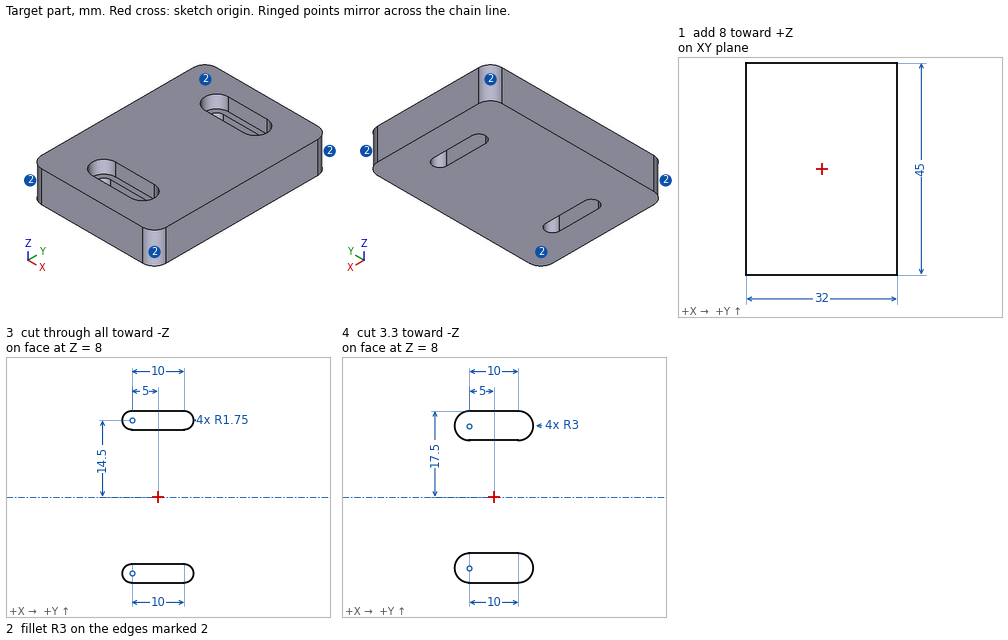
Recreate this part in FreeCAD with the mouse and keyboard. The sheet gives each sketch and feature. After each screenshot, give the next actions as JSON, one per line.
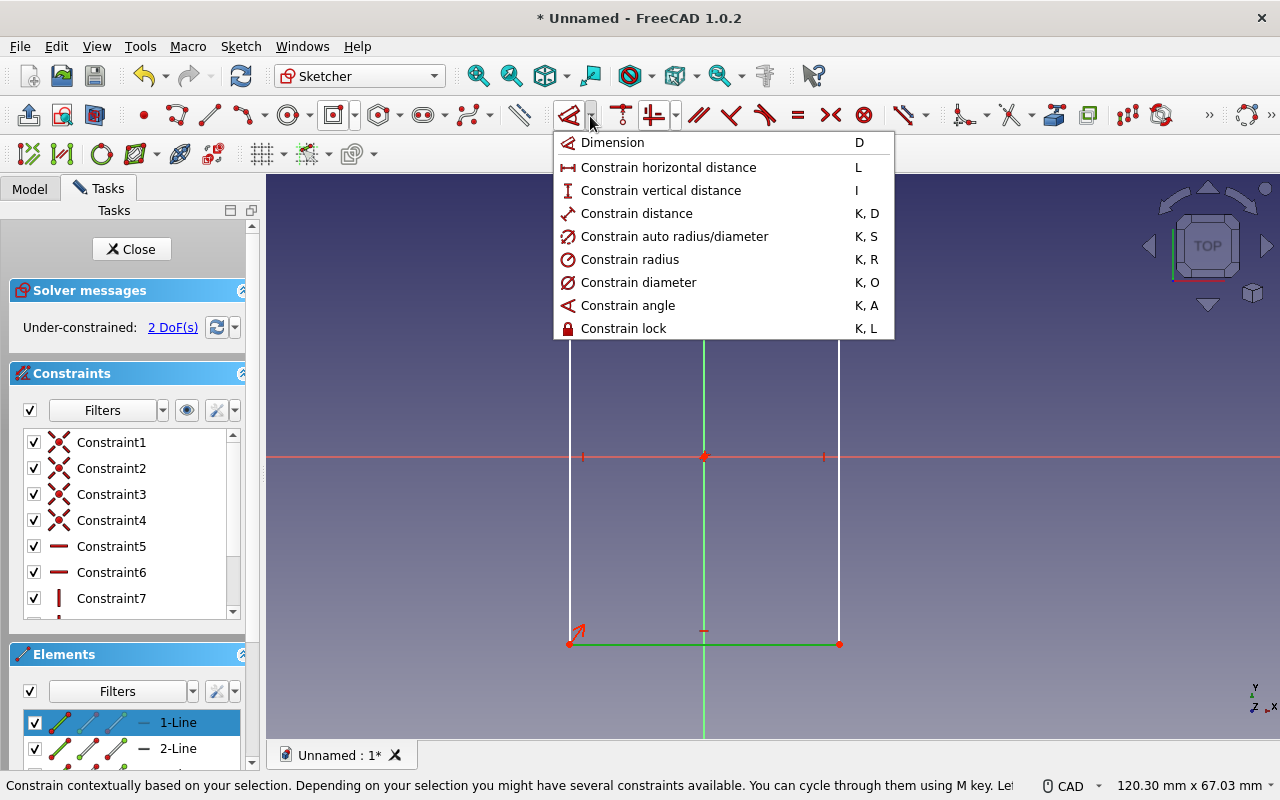
{"action": "left_click", "coordinate": [724, 168]}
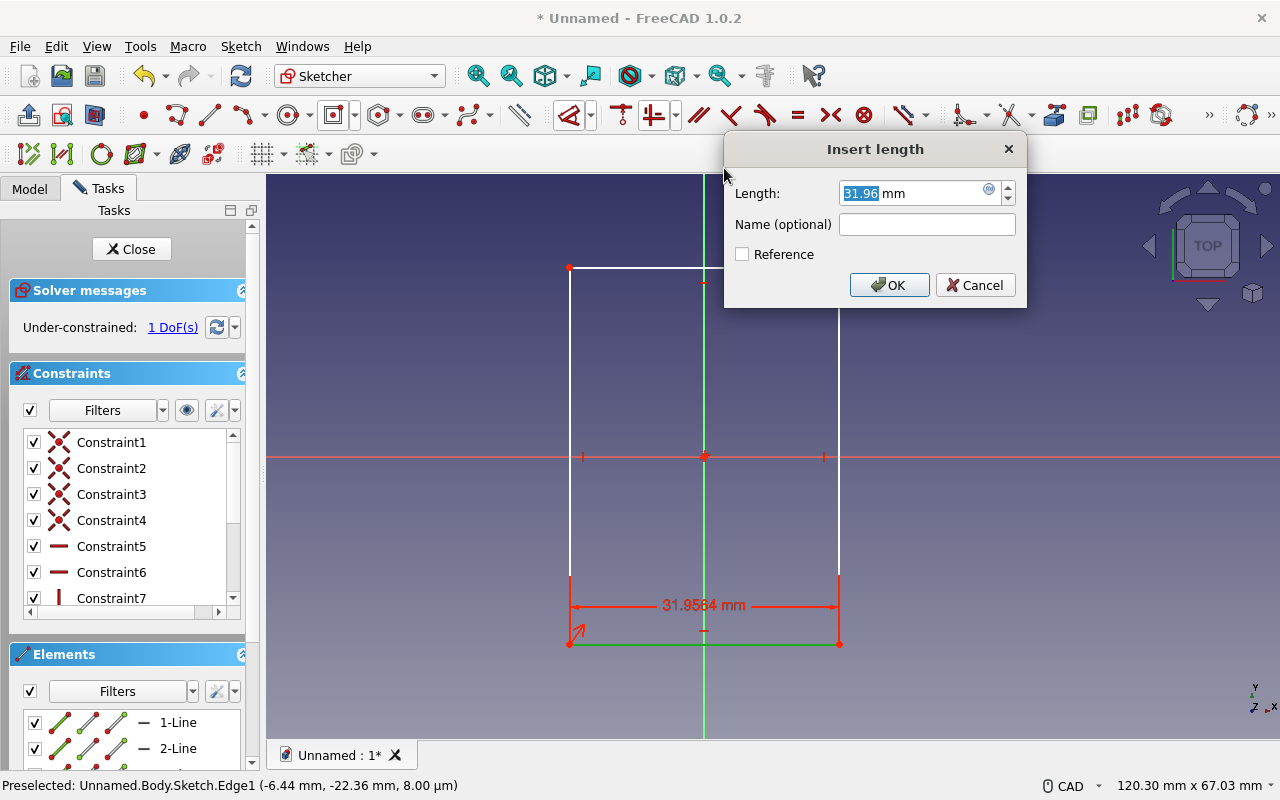
{"action": "type", "text": "32"}
{"action": "key", "text": "Return"}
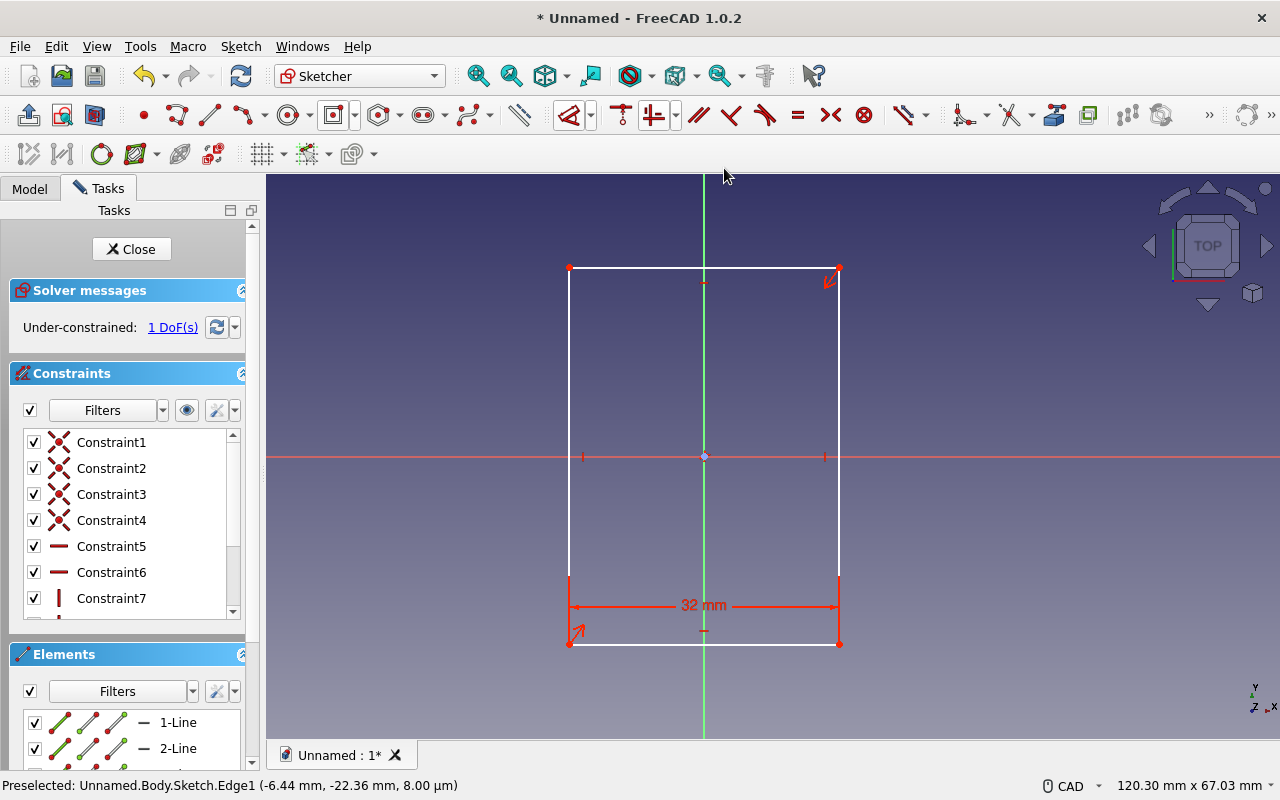
{"action": "left_click", "coordinate": [839, 532]}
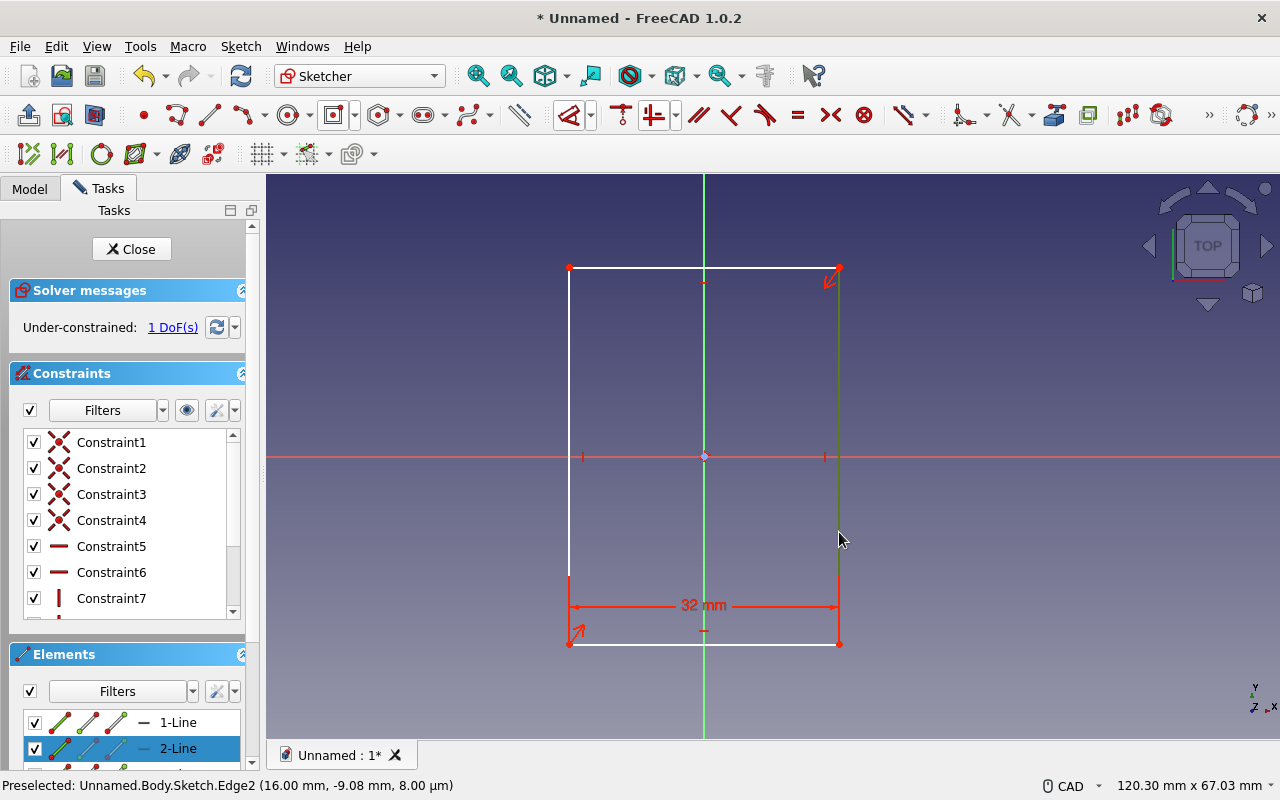
{"action": "left_click", "coordinate": [590, 116]}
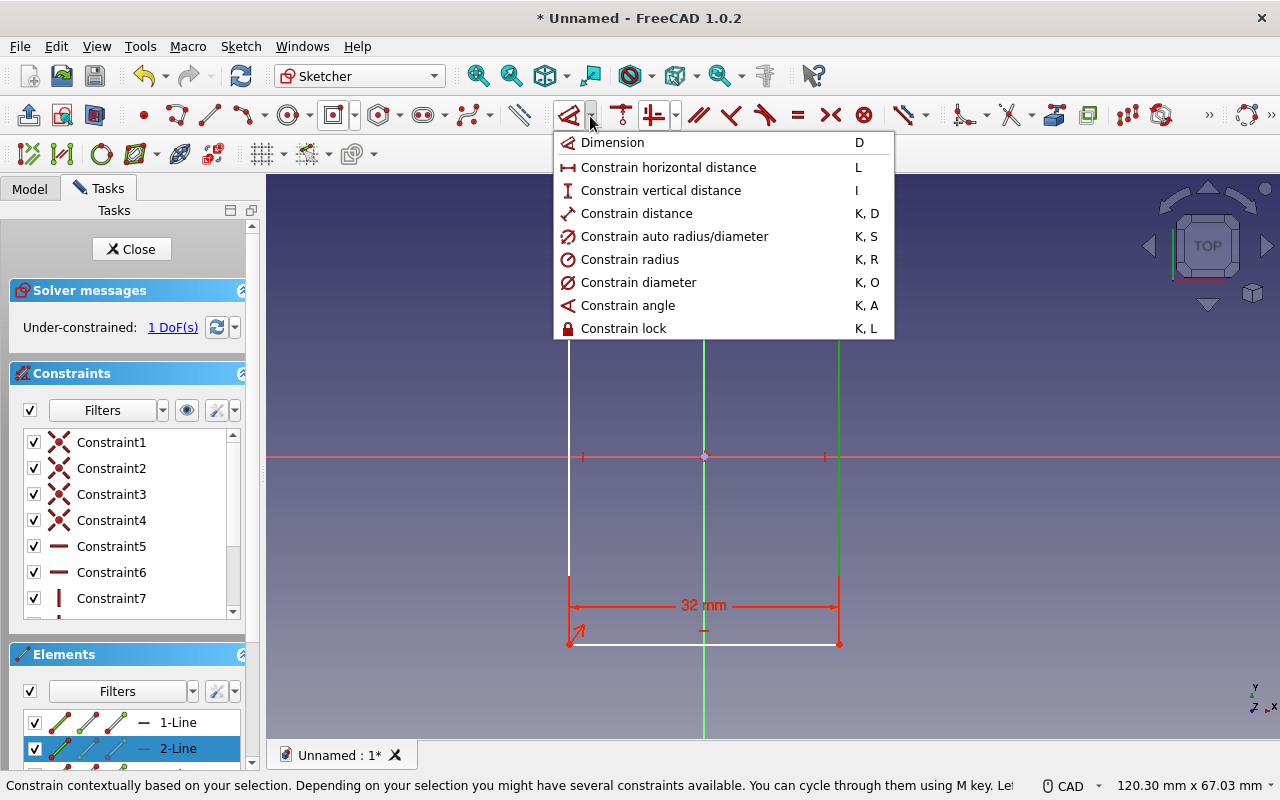
{"action": "left_click", "coordinate": [724, 190]}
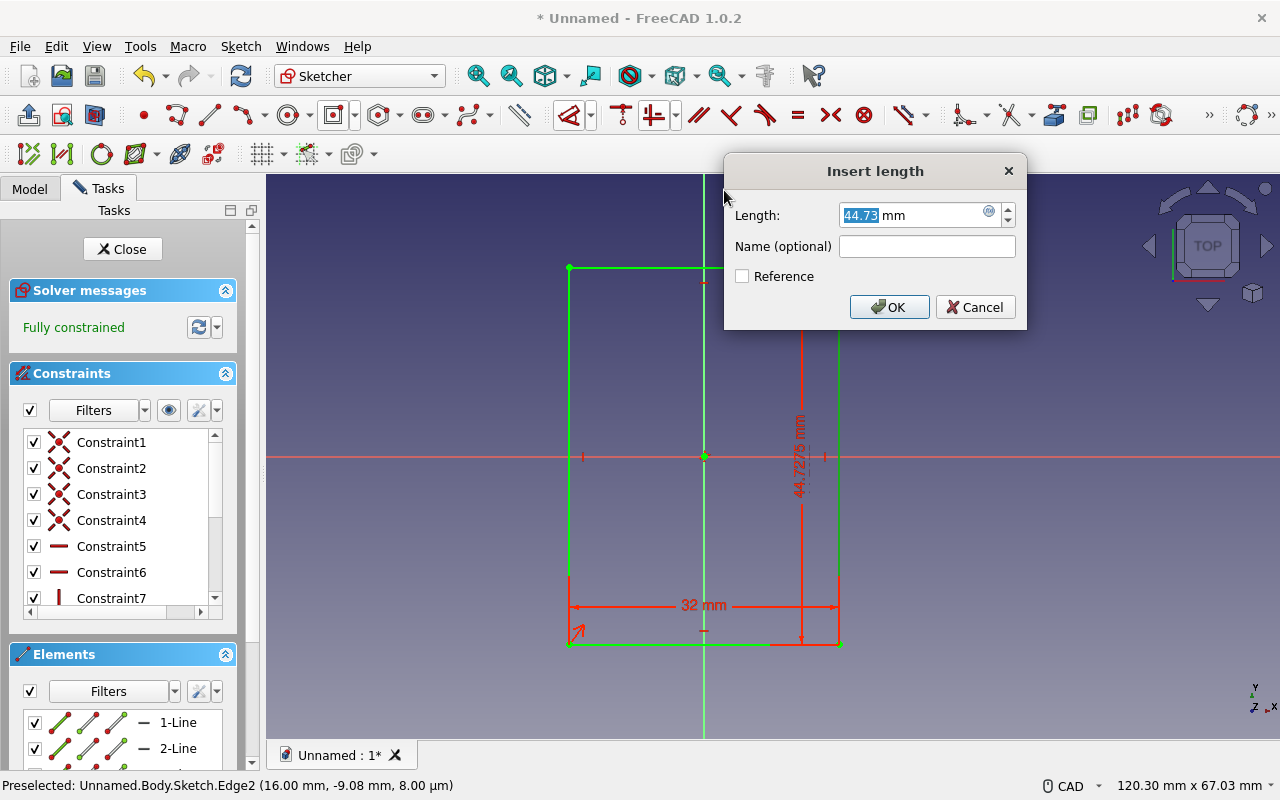
{"action": "type", "text": "45"}
{"action": "key", "text": "Return"}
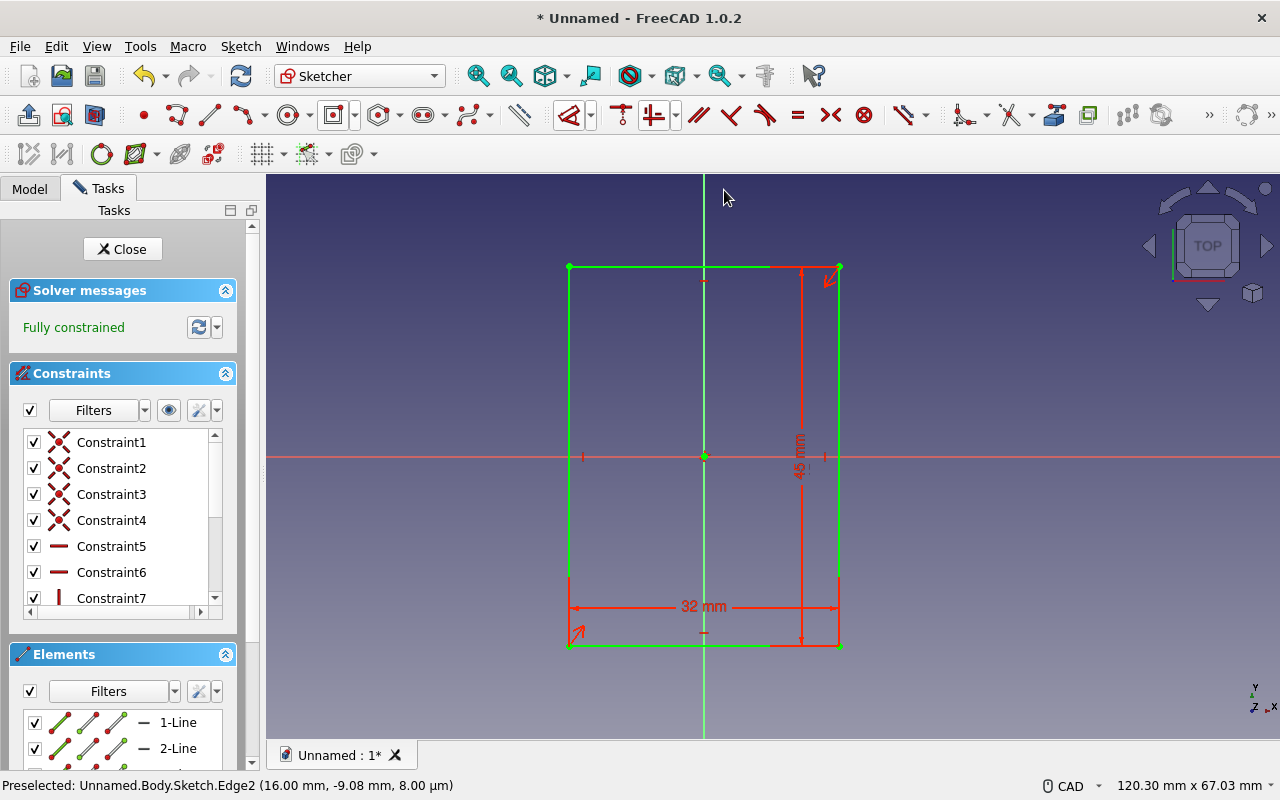
{"action": "left_click", "coordinate": [123, 249]}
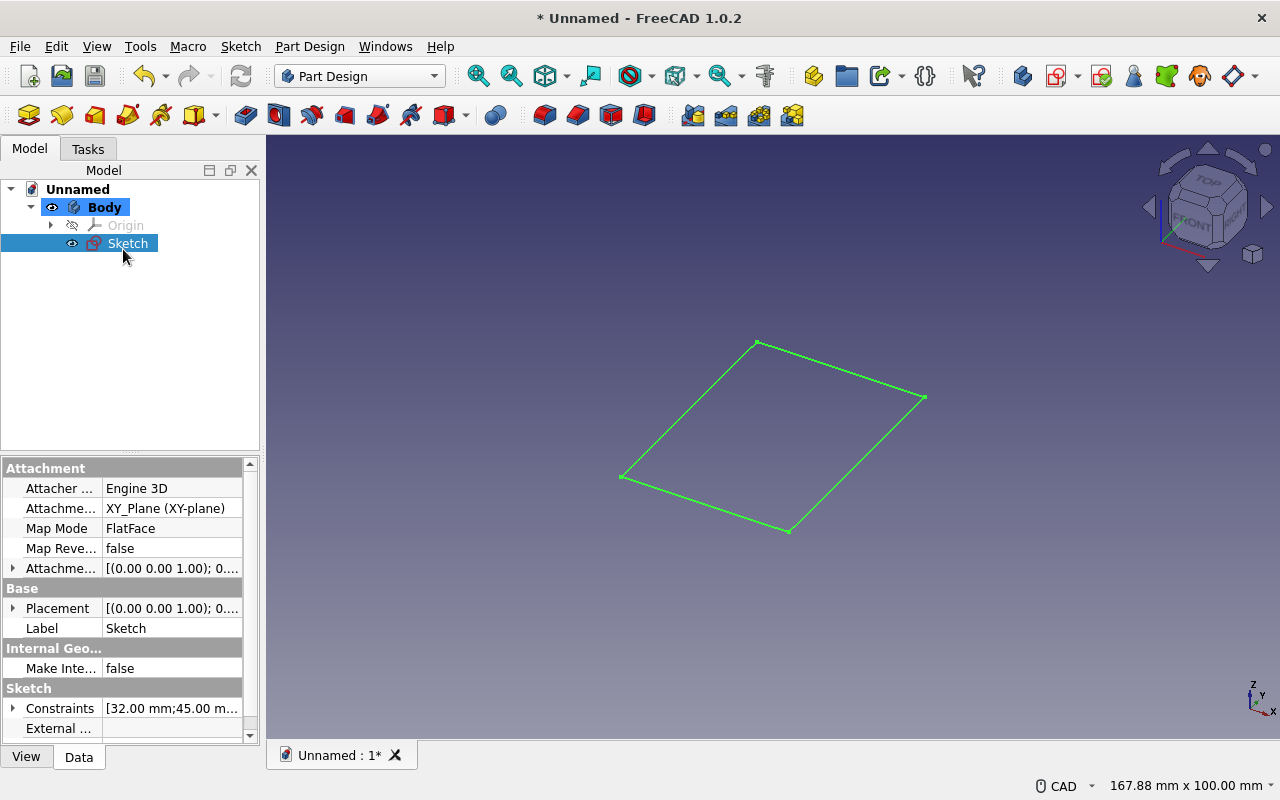
{"action": "left_click", "coordinate": [29, 116]}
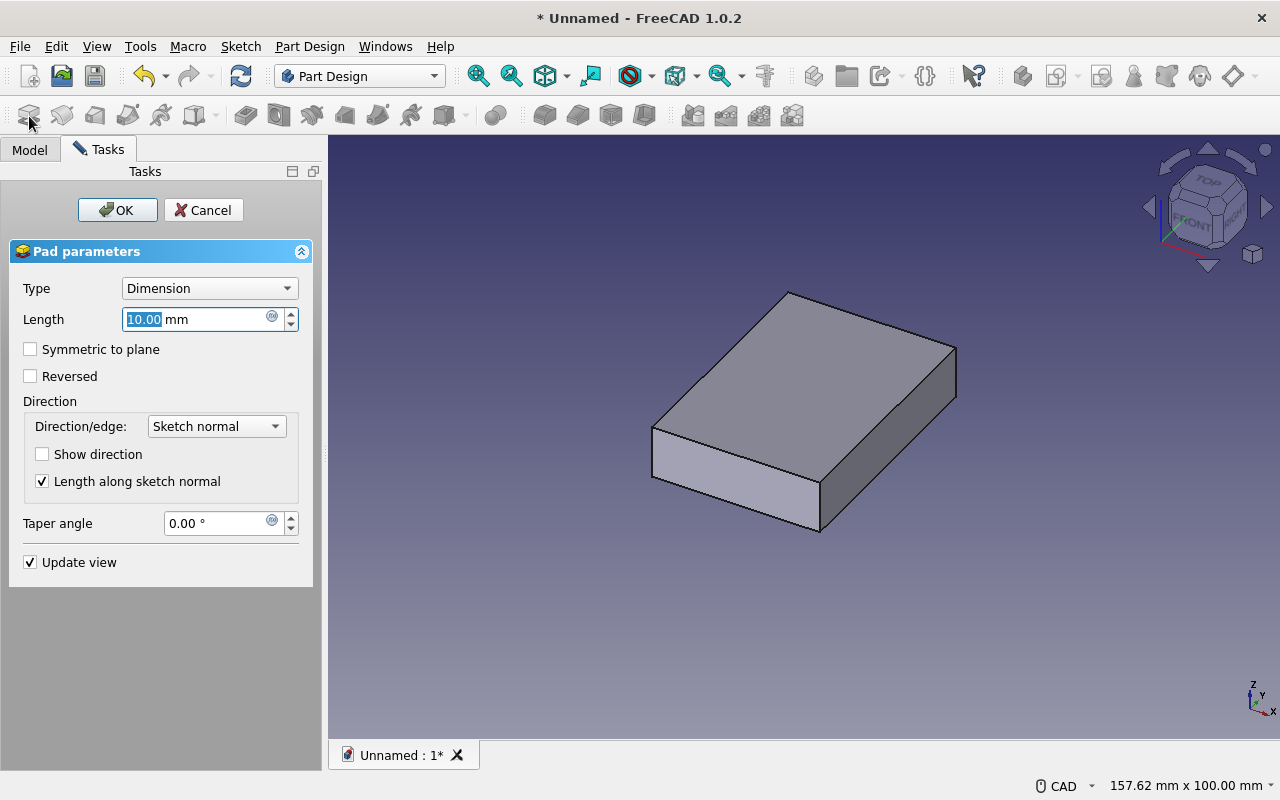
{"action": "type", "text": "8"}
{"action": "key", "text": "Tab"}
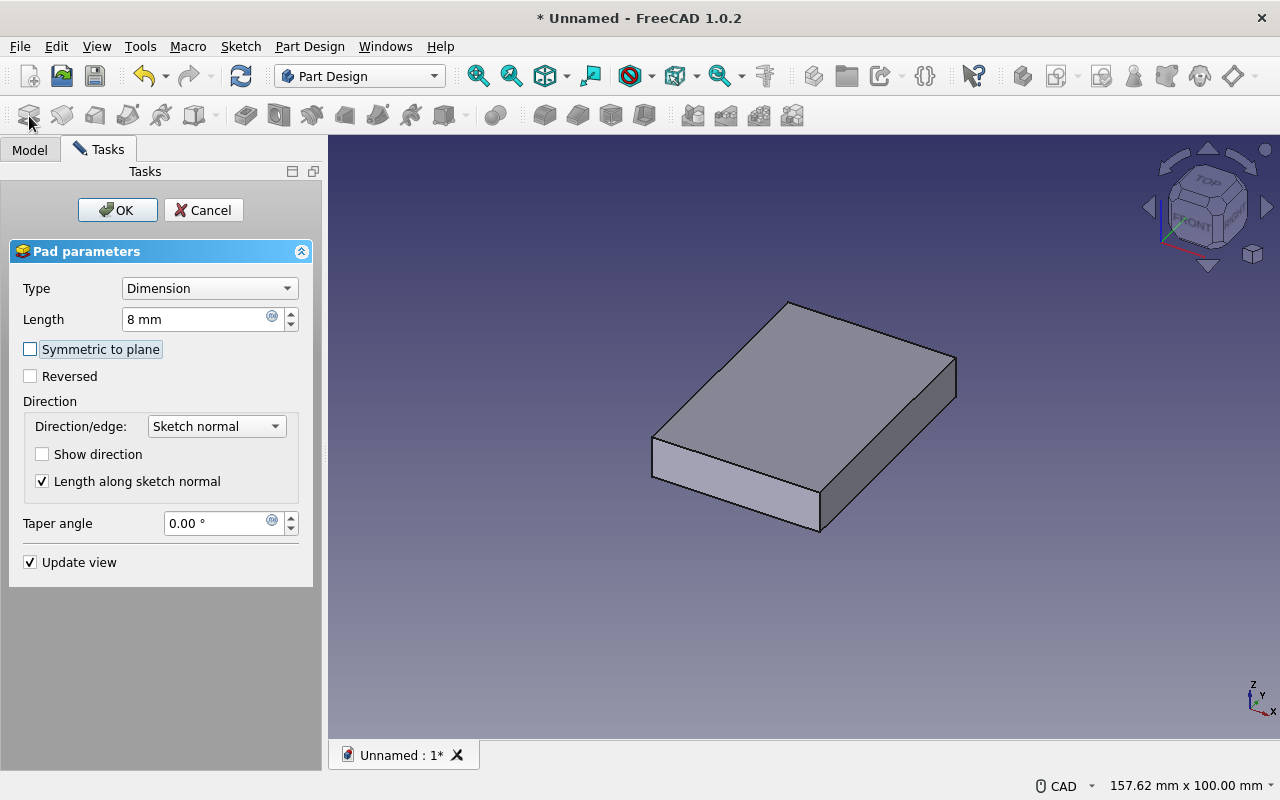
{"action": "left_click", "coordinate": [118, 210]}